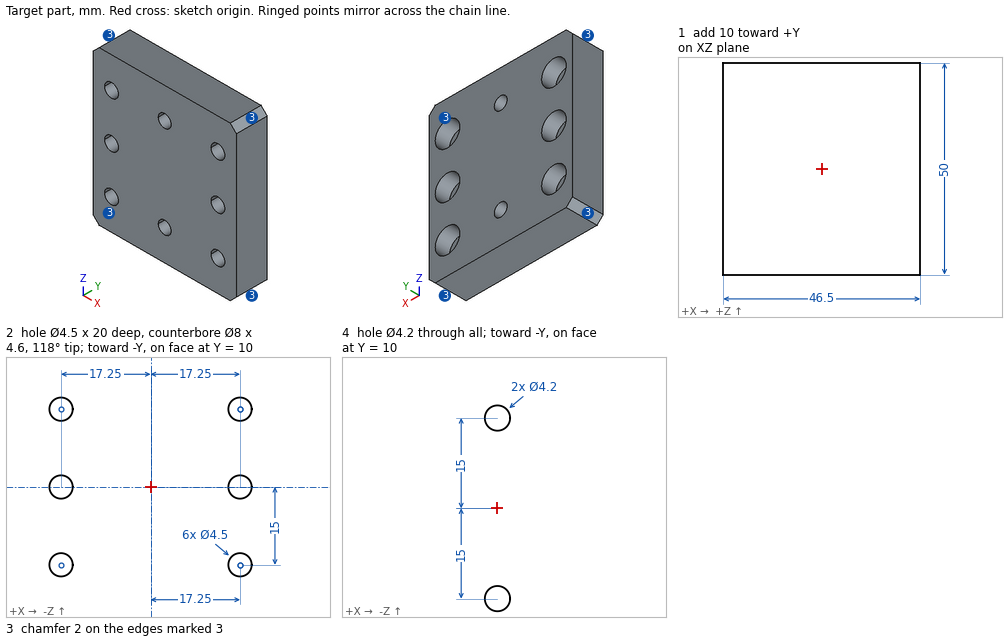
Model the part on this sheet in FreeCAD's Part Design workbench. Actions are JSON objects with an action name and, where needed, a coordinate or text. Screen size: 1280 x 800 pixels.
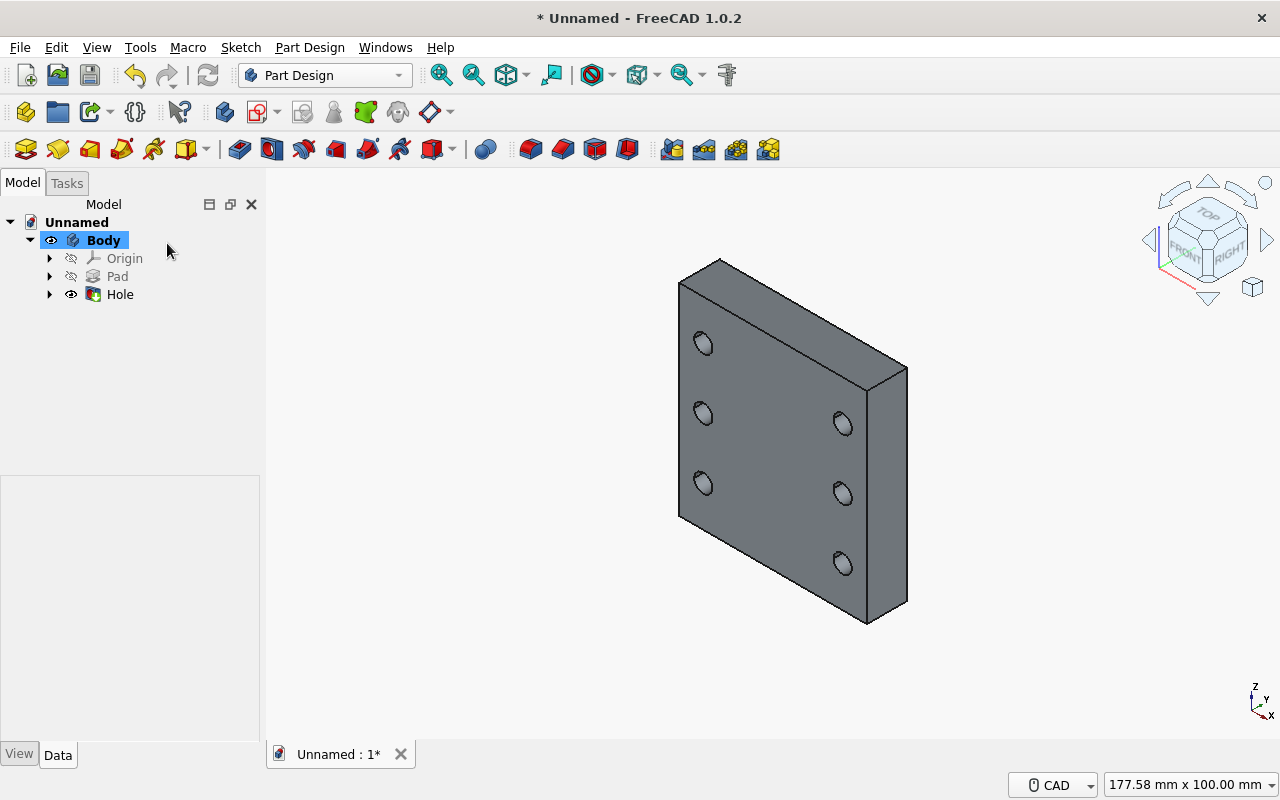
{"action": "left_click", "coordinate": [887, 378]}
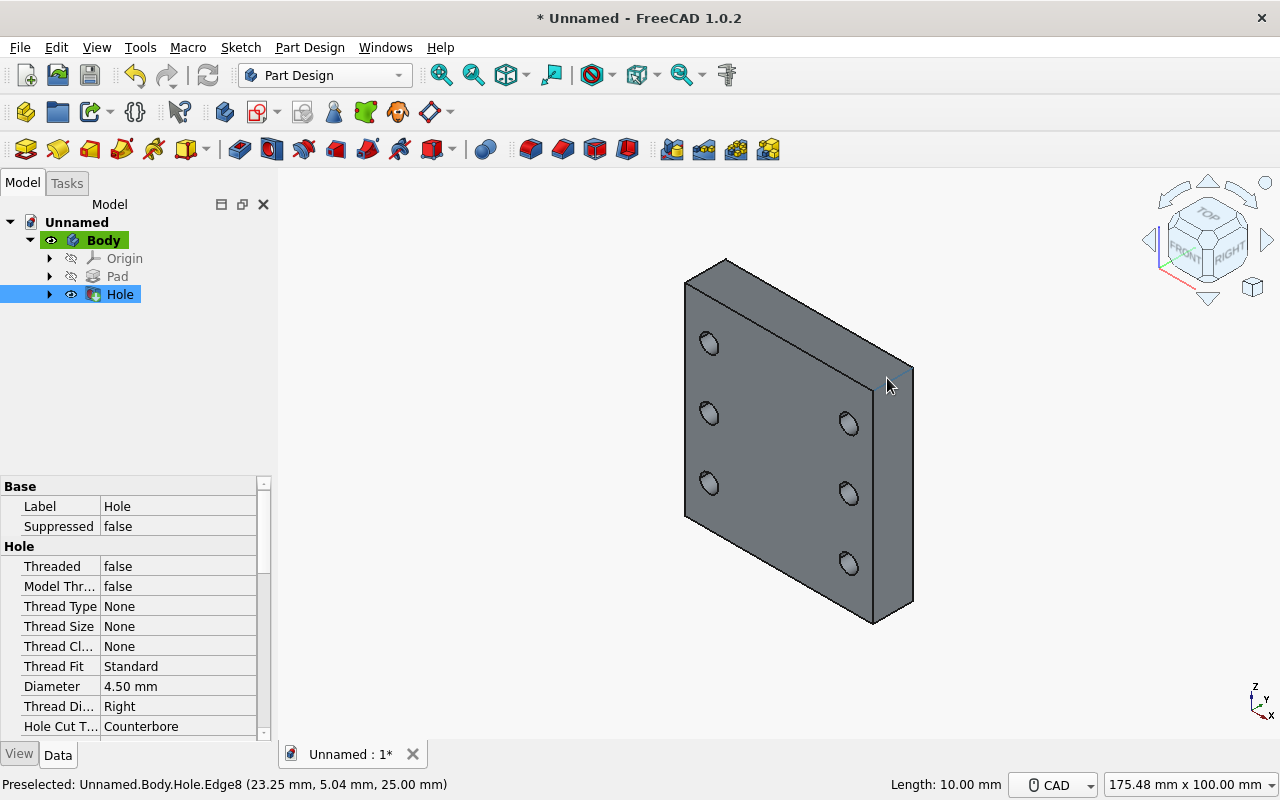
{"action": "key", "text": "2"}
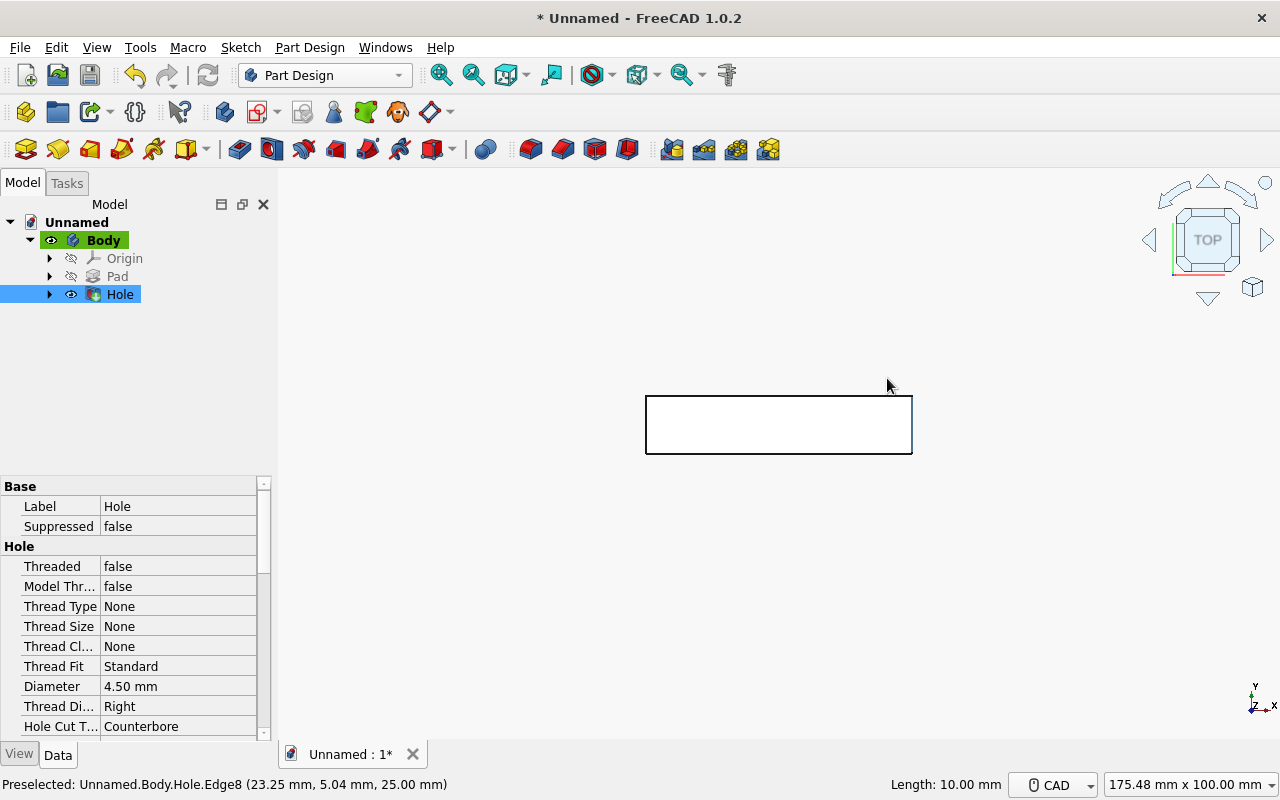
{"action": "left_click", "coordinate": [442, 76]}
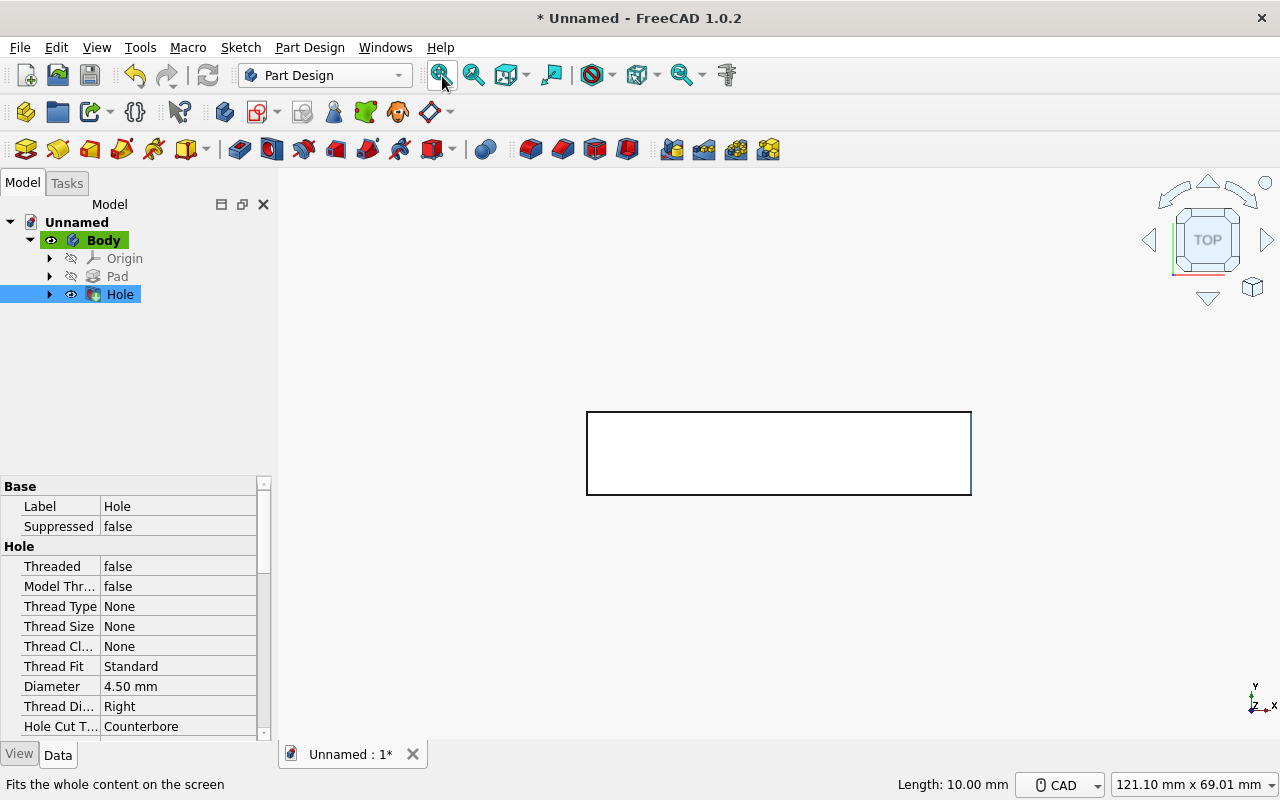
{"action": "left_click", "coordinate": [587, 452], "text": "ctrl"}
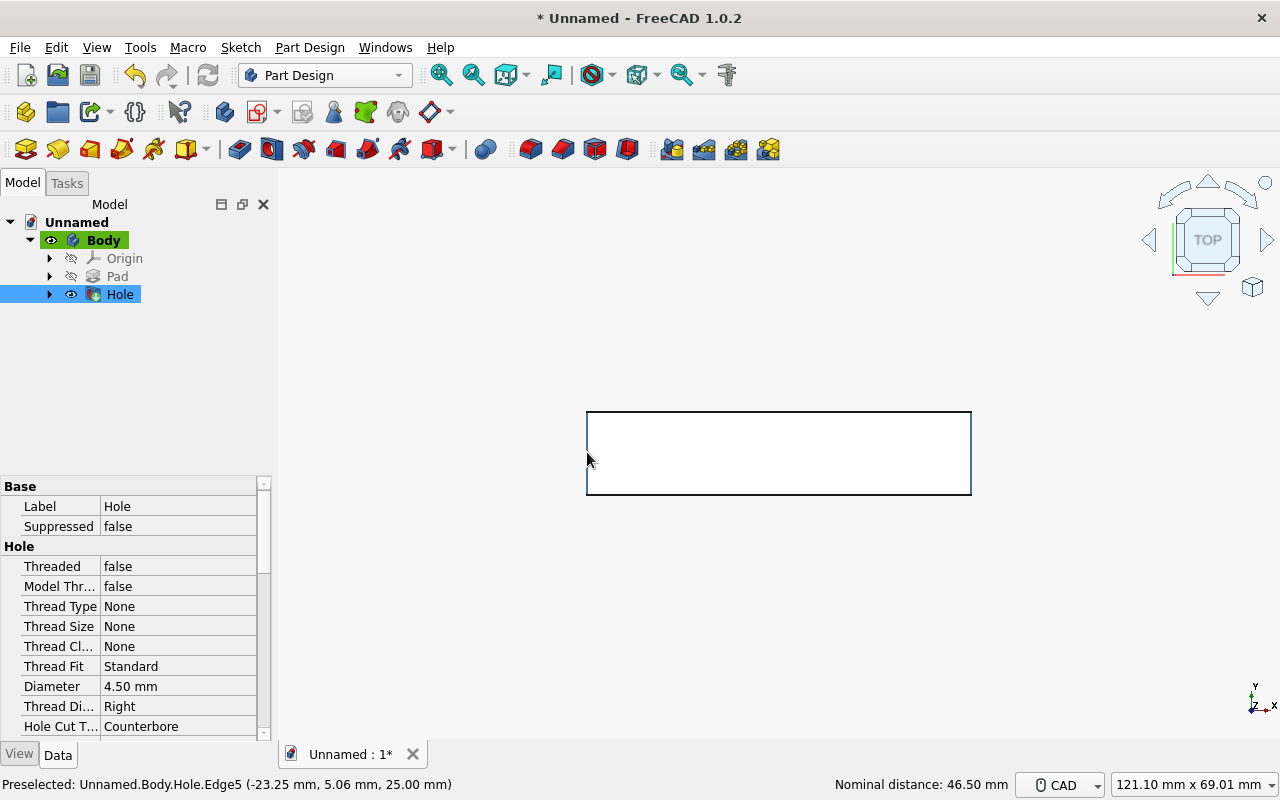
{"action": "key", "text": "1"}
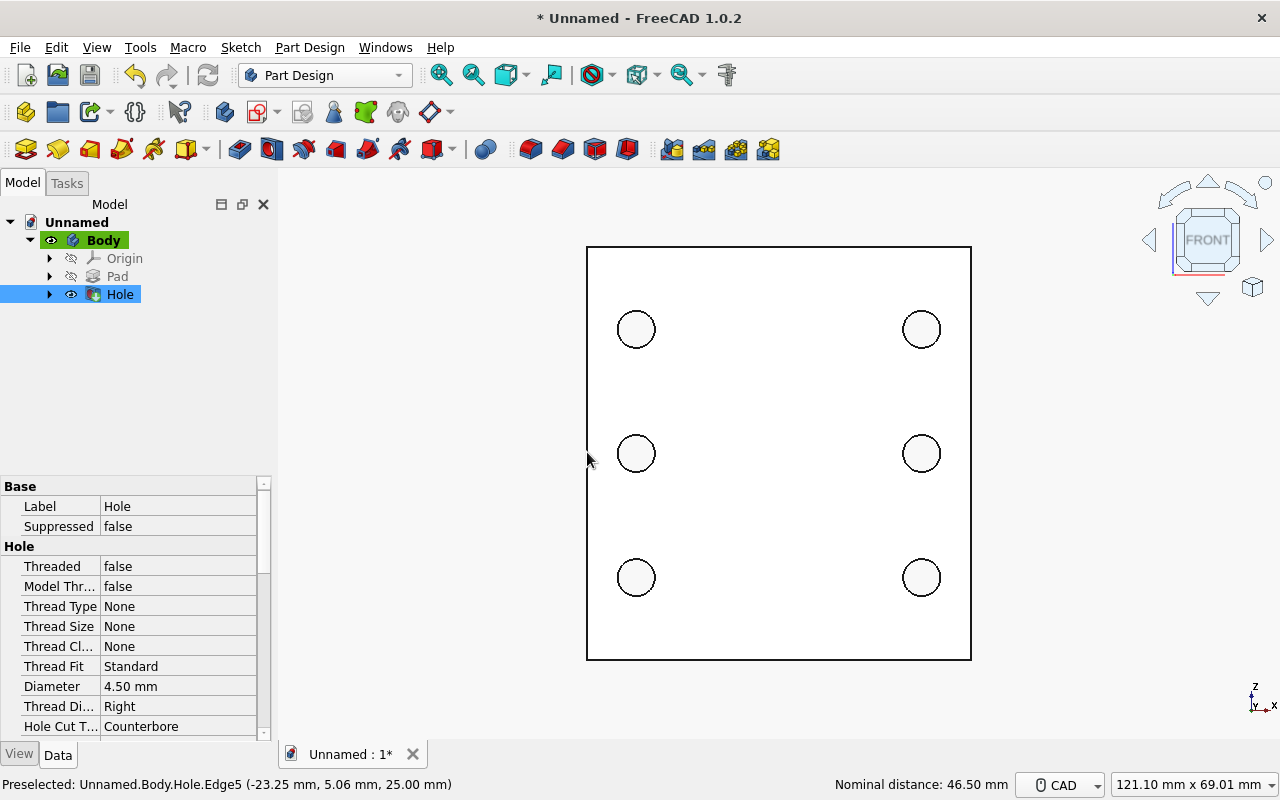
{"action": "key", "text": "3"}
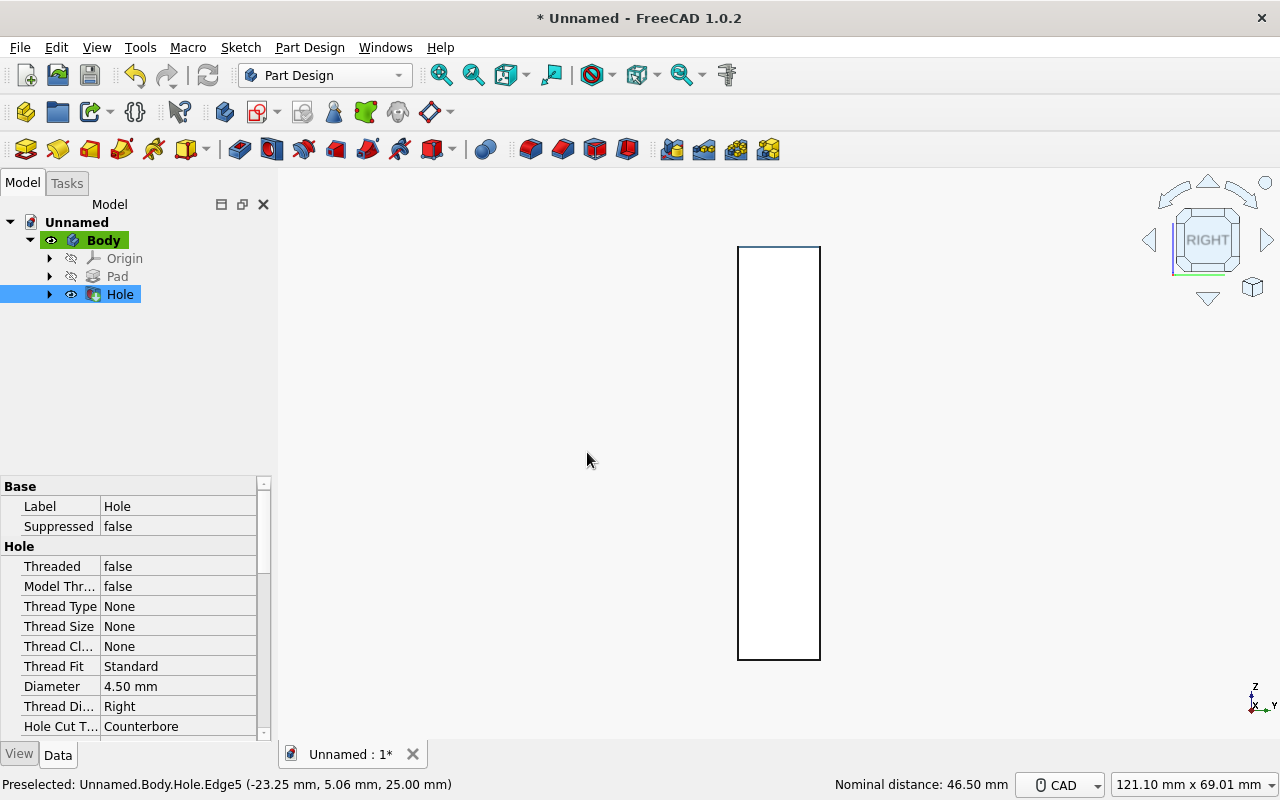
{"action": "left_click", "coordinate": [779, 659], "text": "ctrl"}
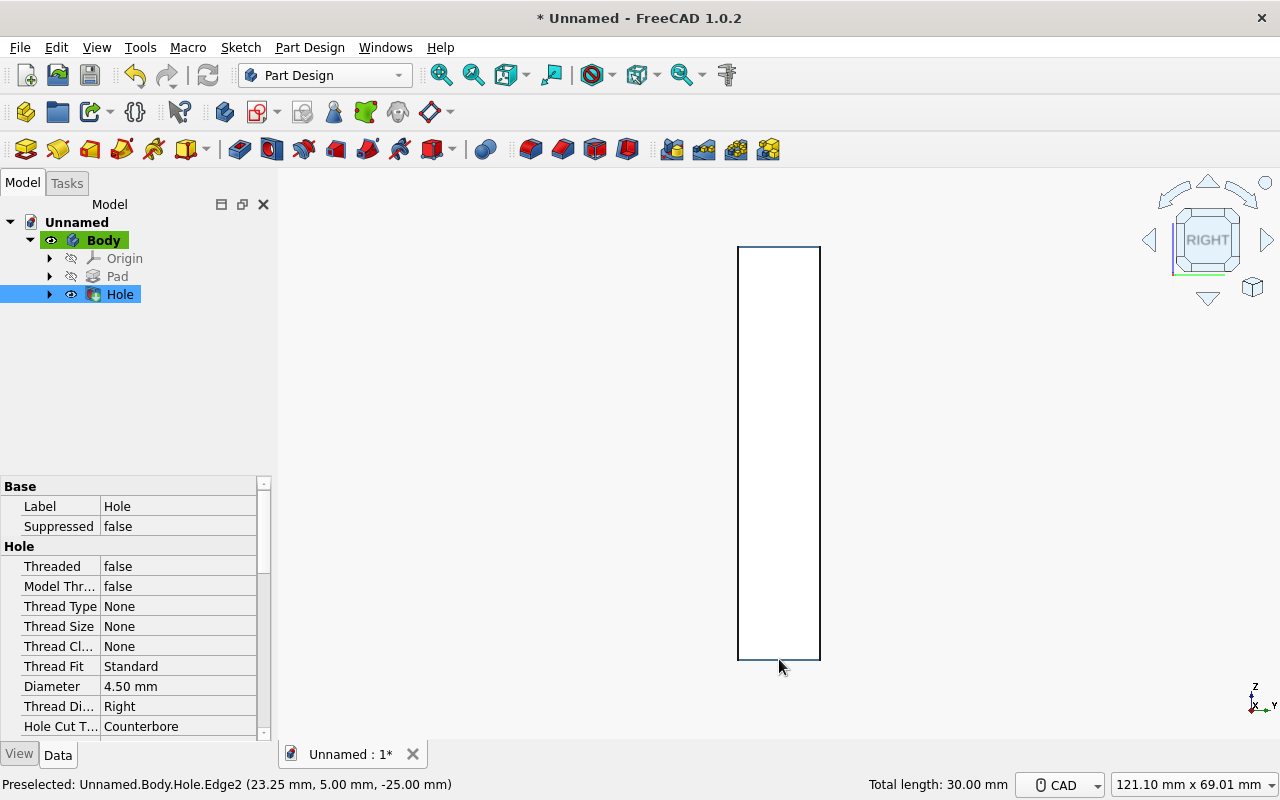
{"action": "key", "text": "5"}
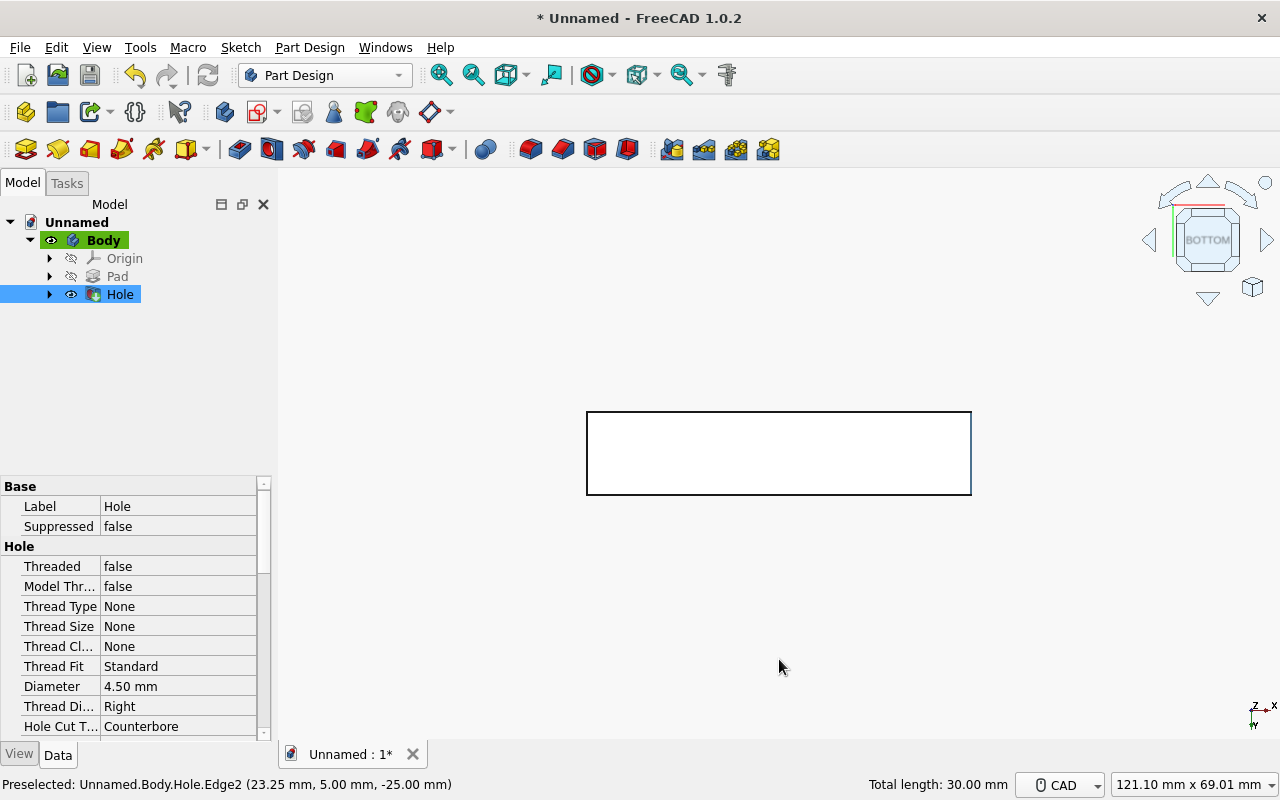
{"action": "left_click", "coordinate": [442, 76]}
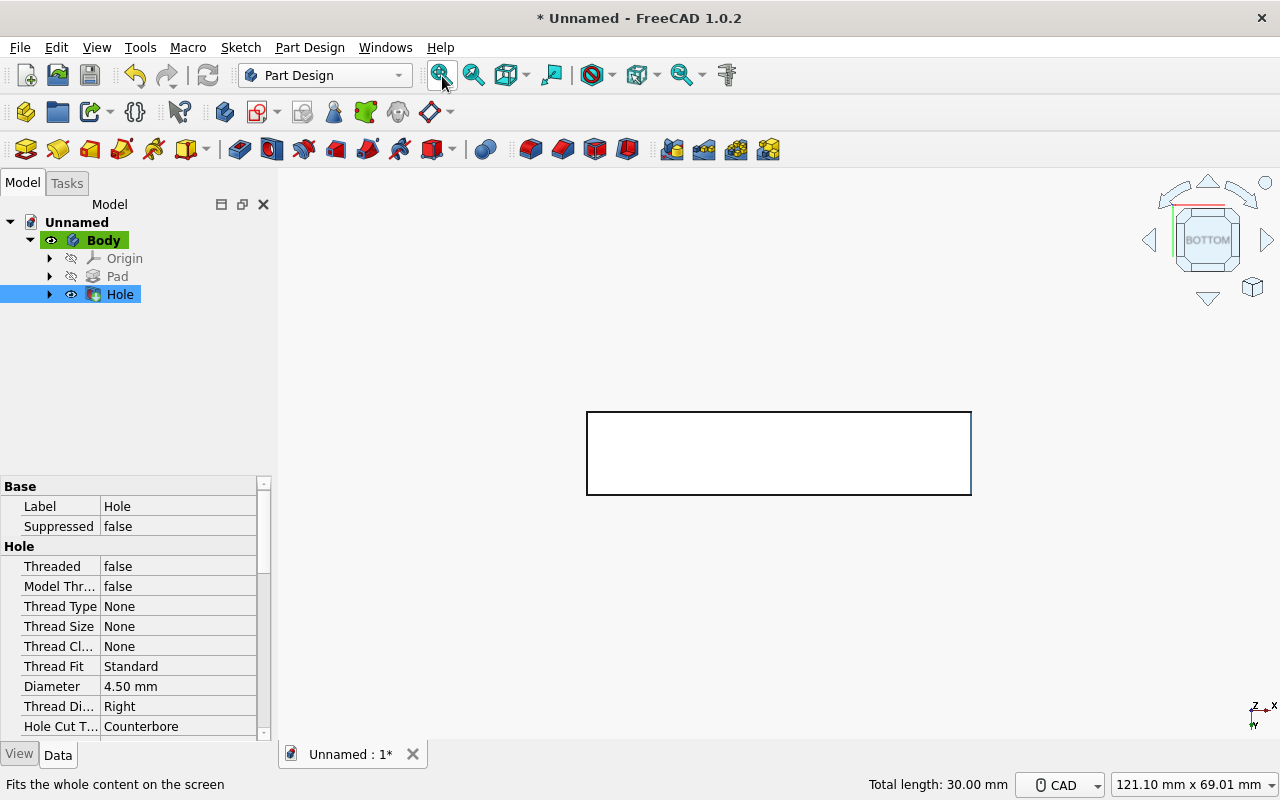
{"action": "left_click", "coordinate": [587, 452], "text": "ctrl"}